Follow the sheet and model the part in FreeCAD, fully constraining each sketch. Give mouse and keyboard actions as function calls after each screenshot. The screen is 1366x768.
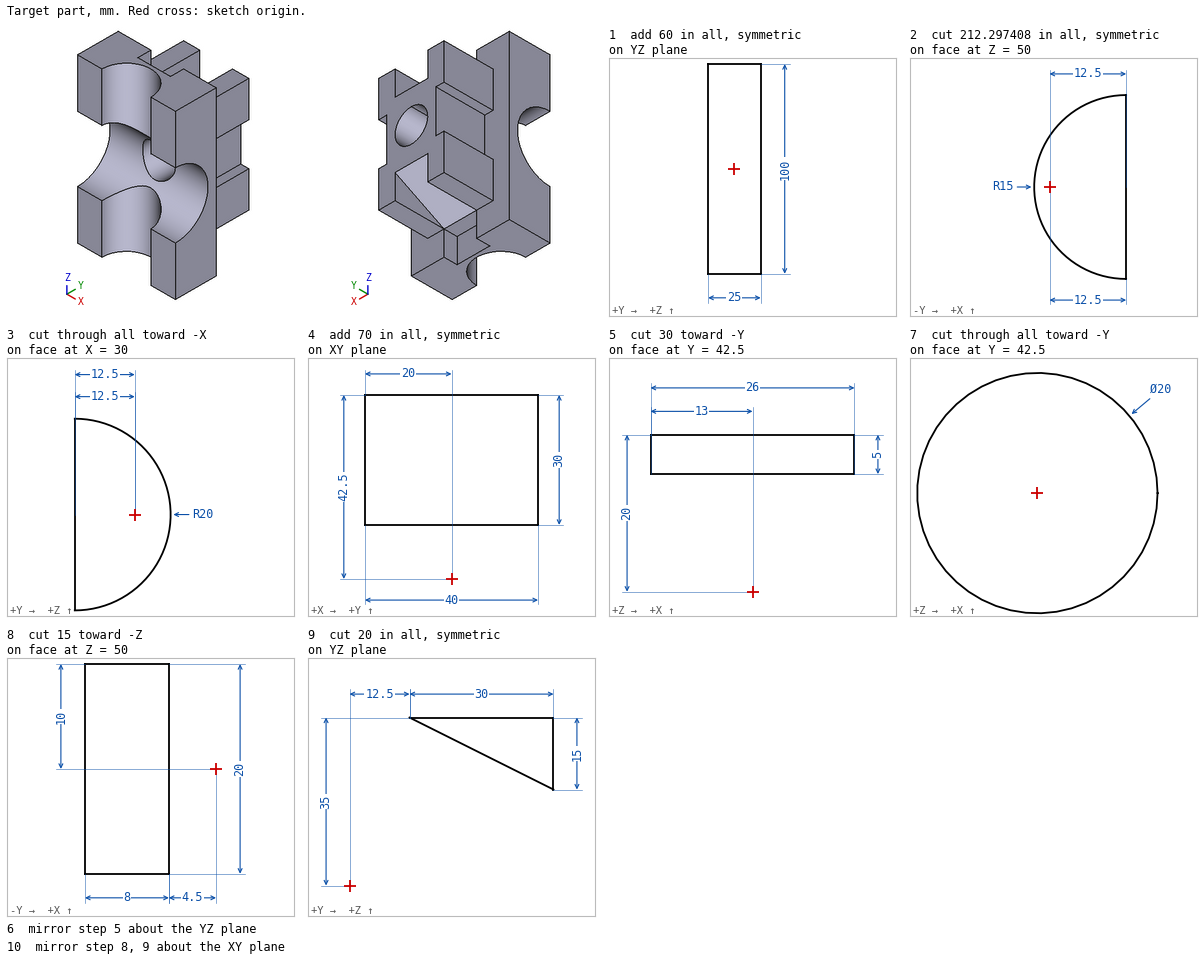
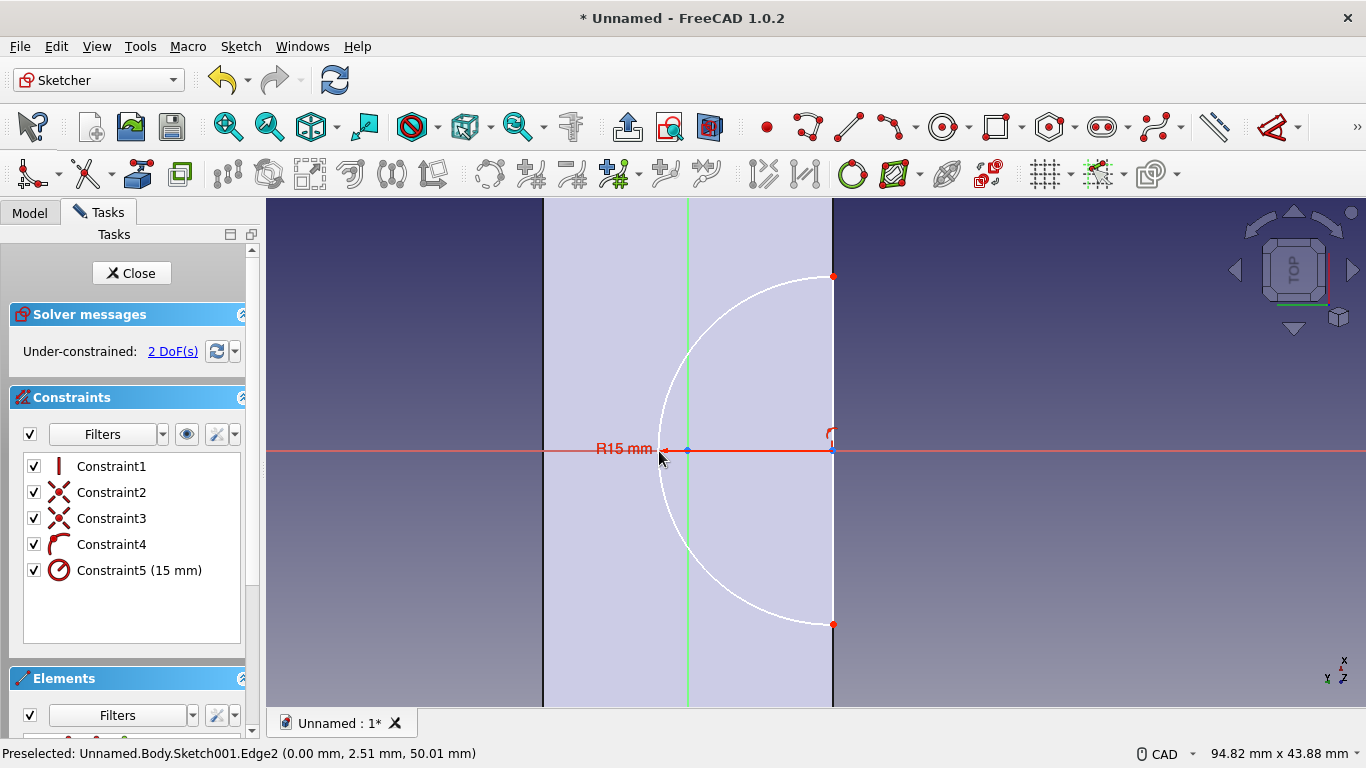
click(833, 625)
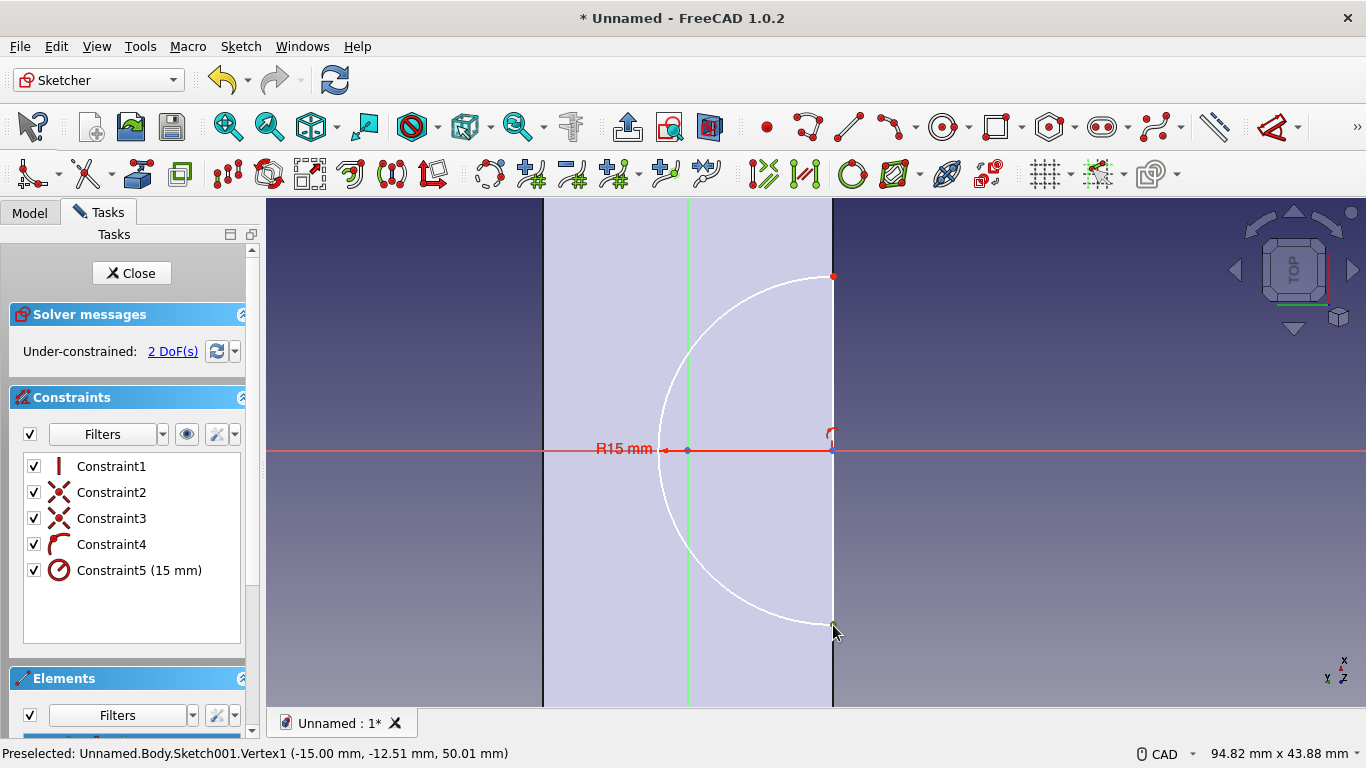
key(l)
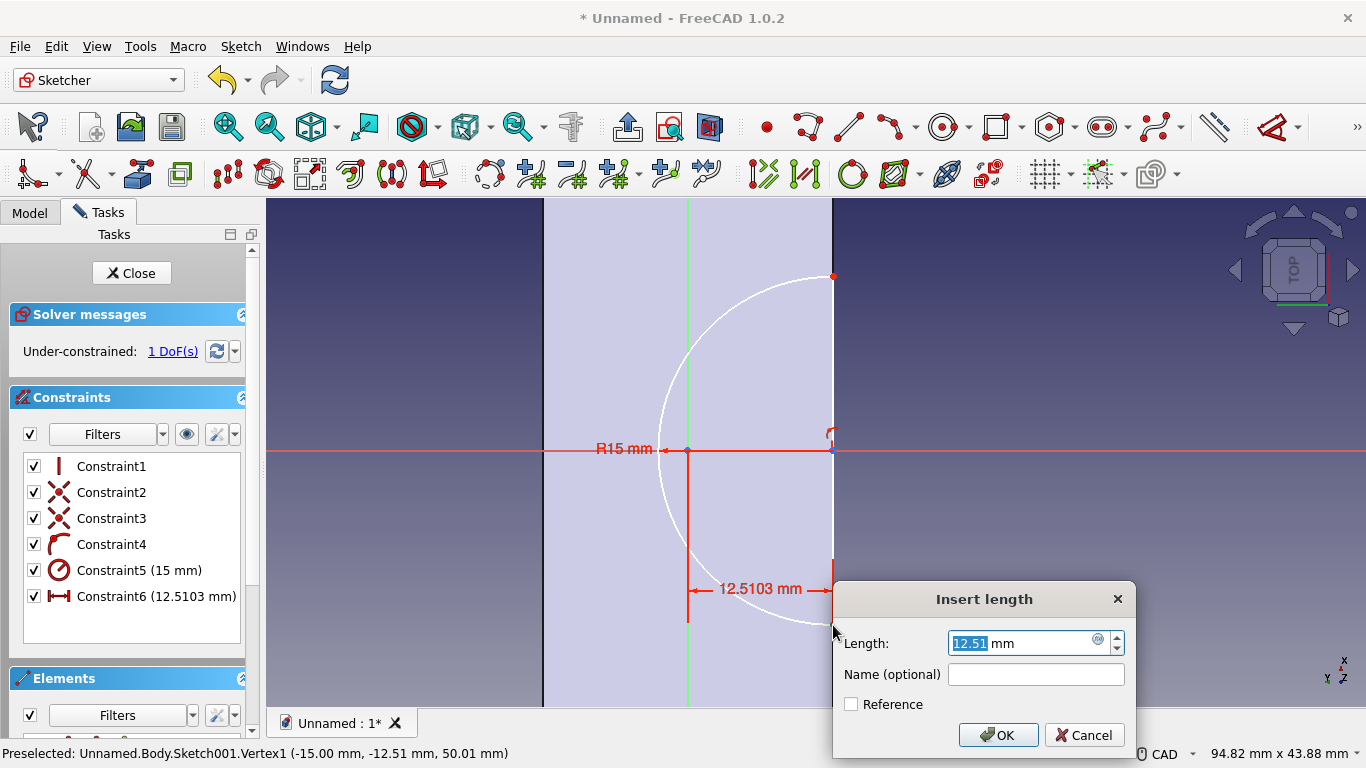
text(12.5)
key(Return)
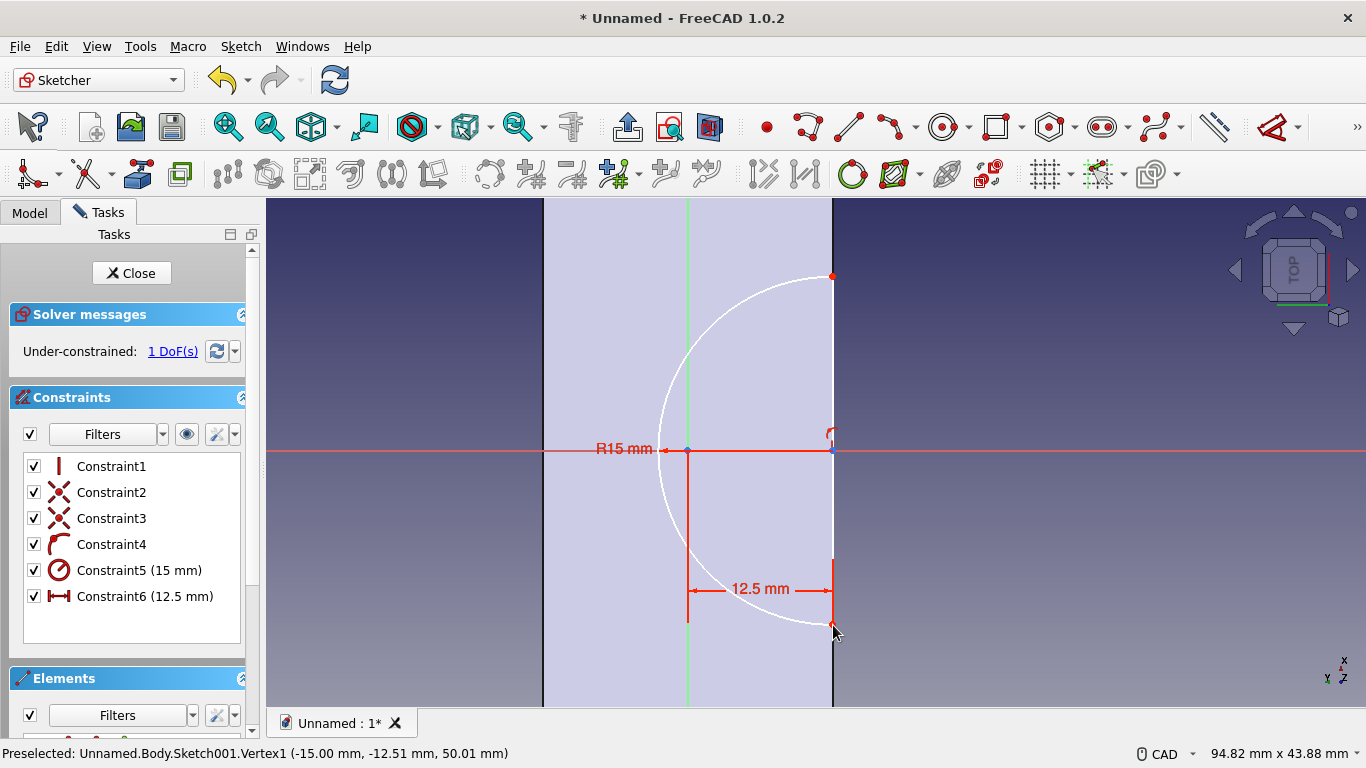
click(832, 451)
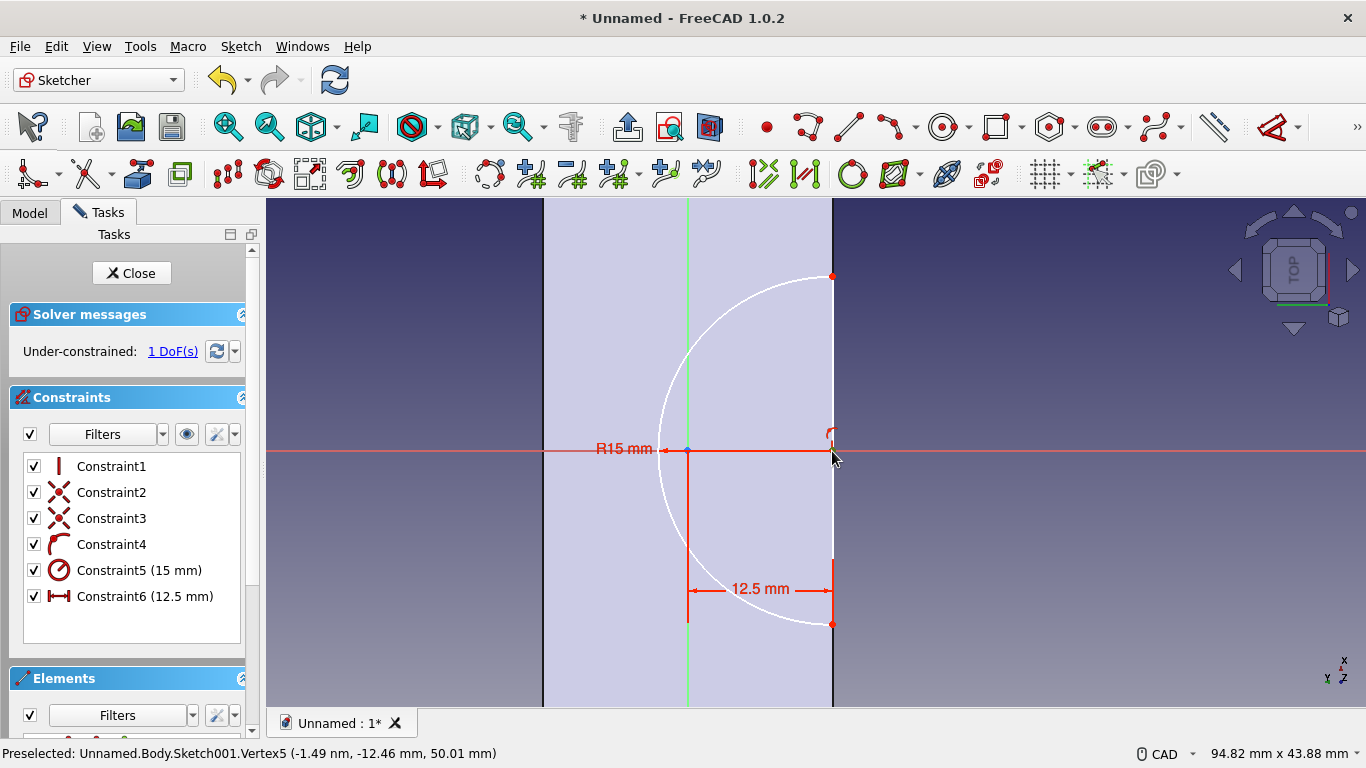
key(l)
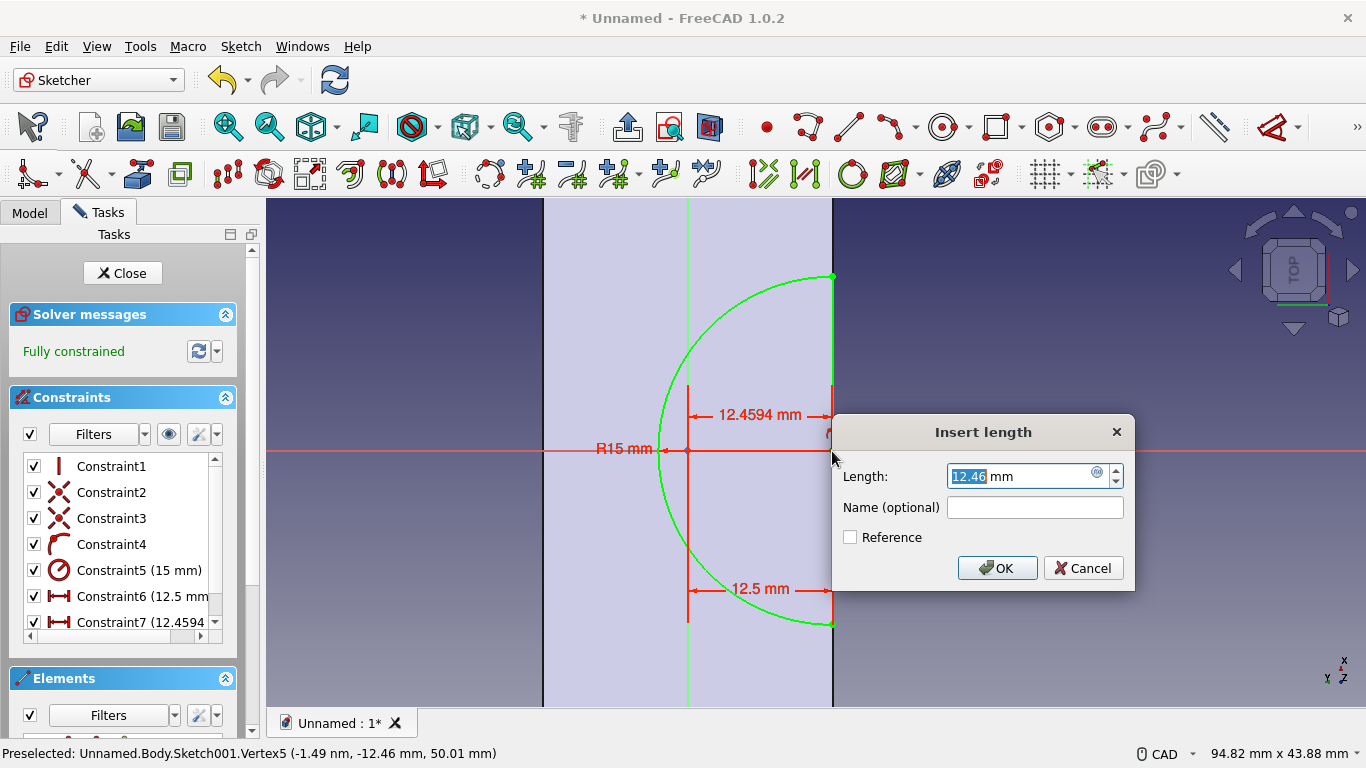
text(12.5)
key(Return)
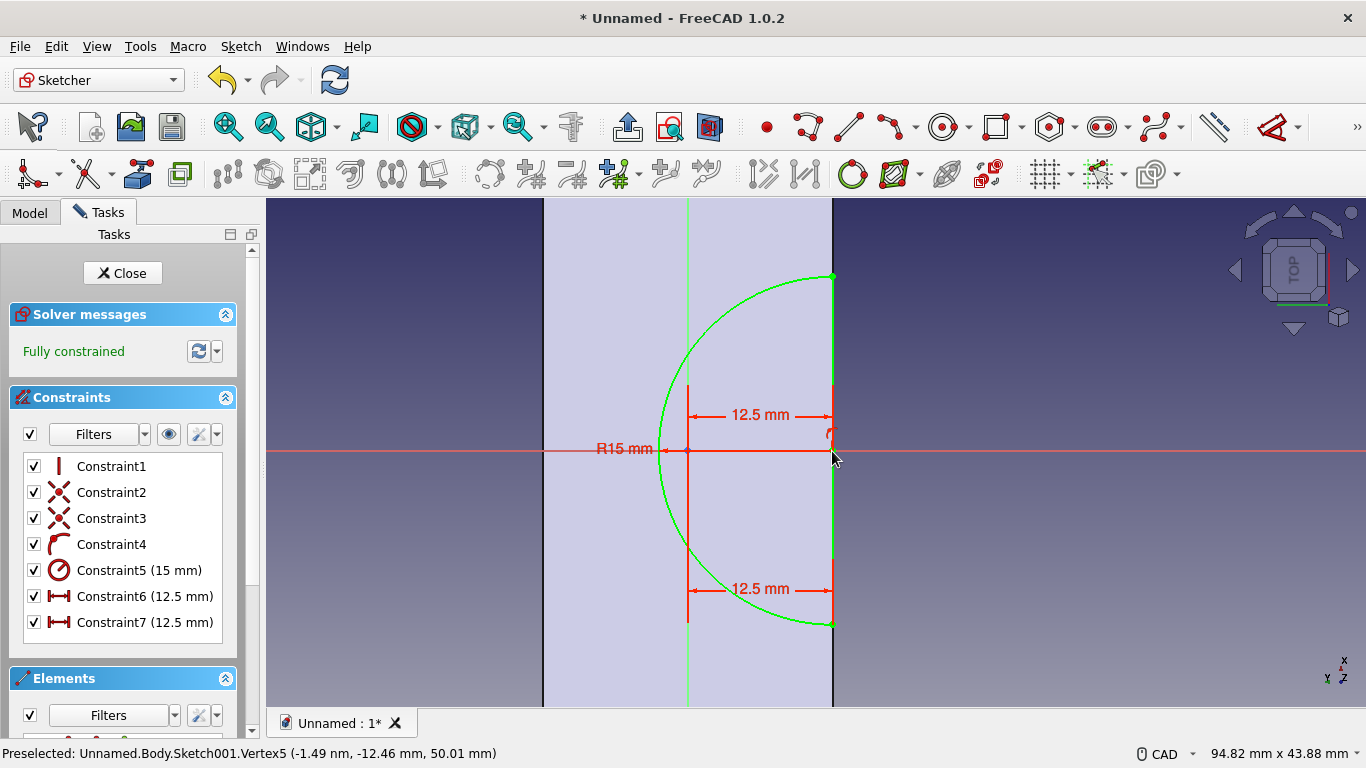
click(123, 273)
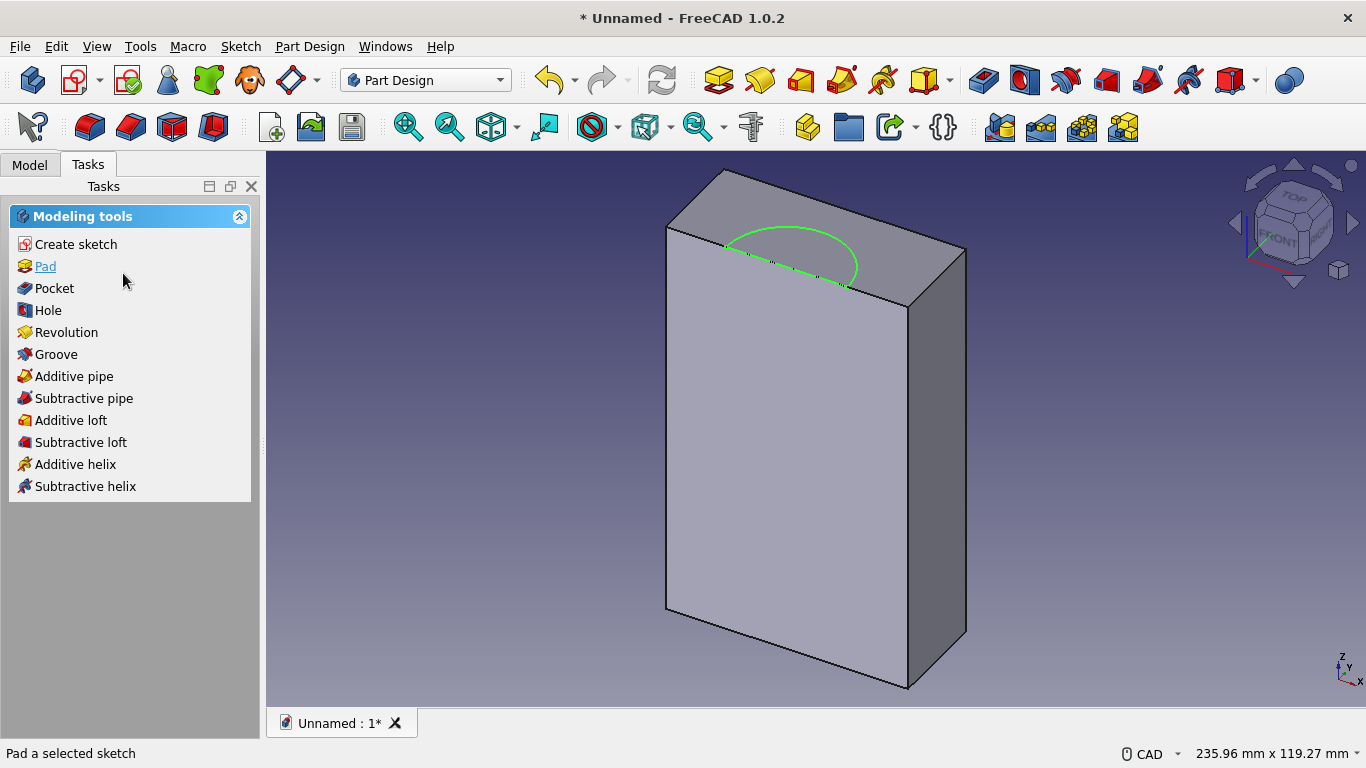
click(984, 80)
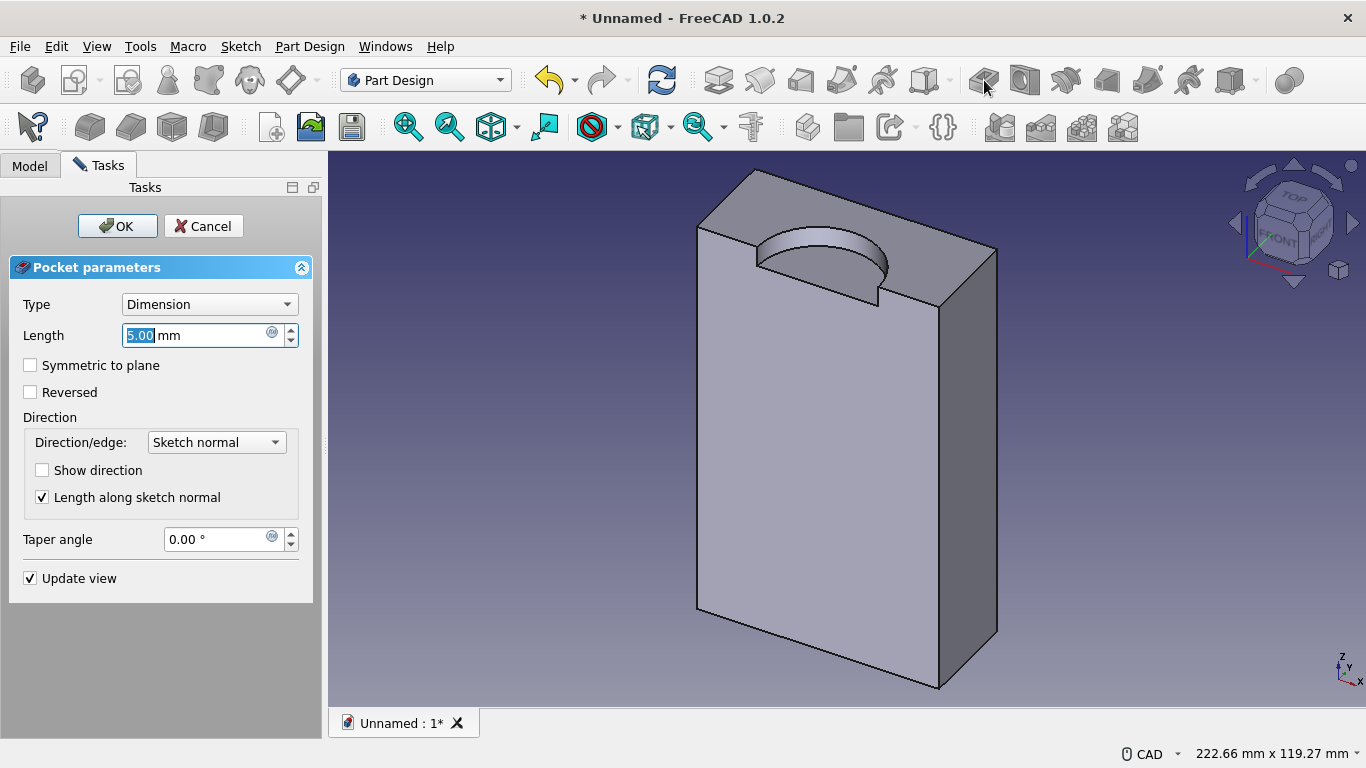
text(212.297408)
key(Tab)